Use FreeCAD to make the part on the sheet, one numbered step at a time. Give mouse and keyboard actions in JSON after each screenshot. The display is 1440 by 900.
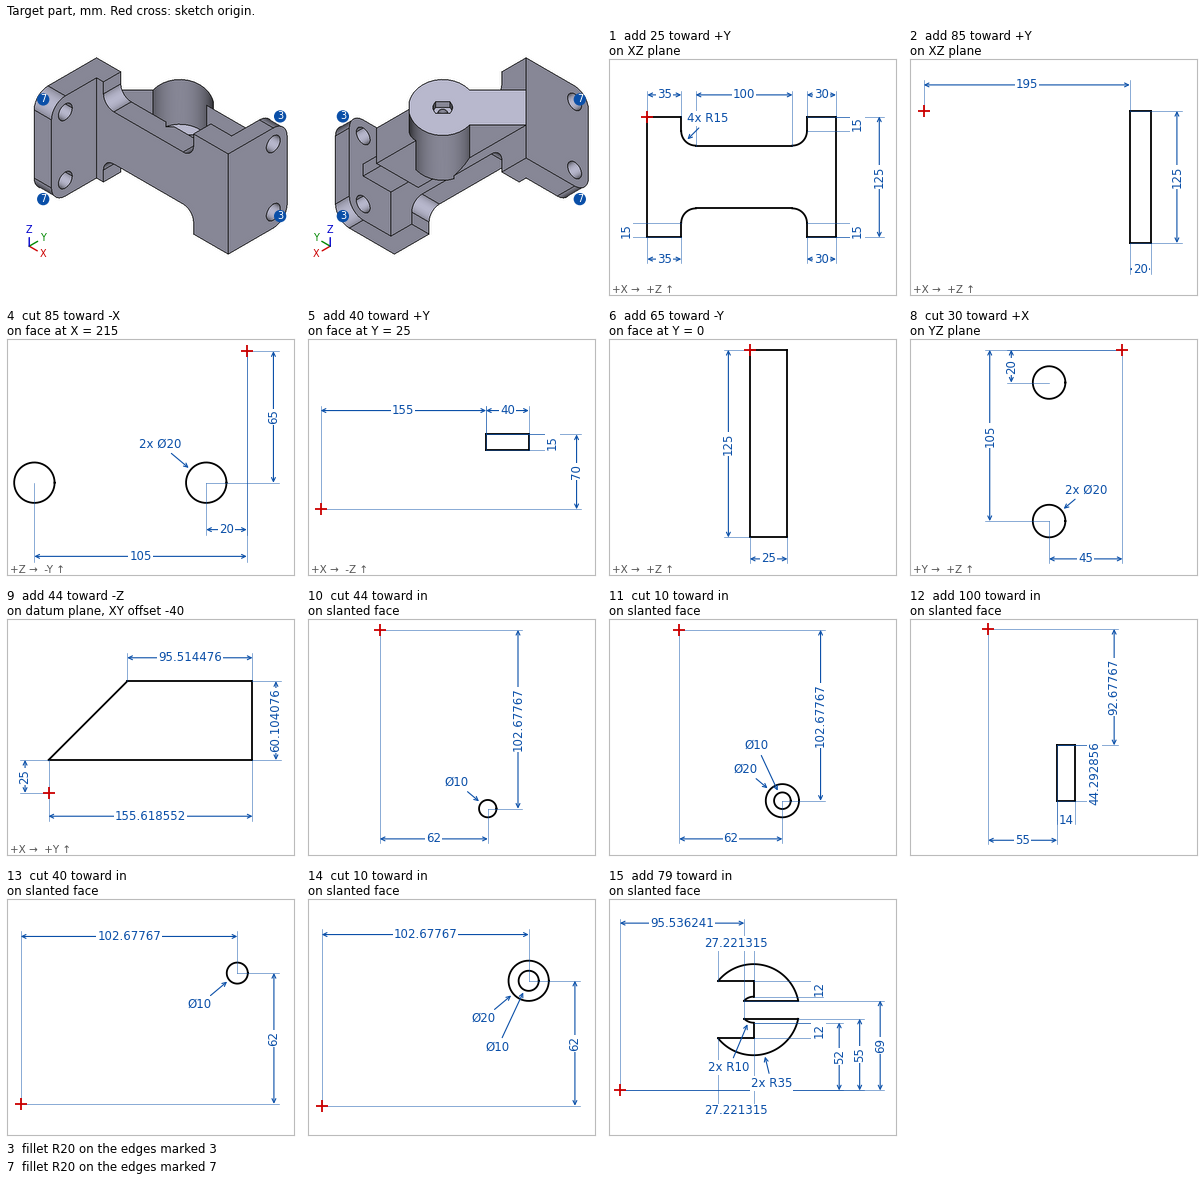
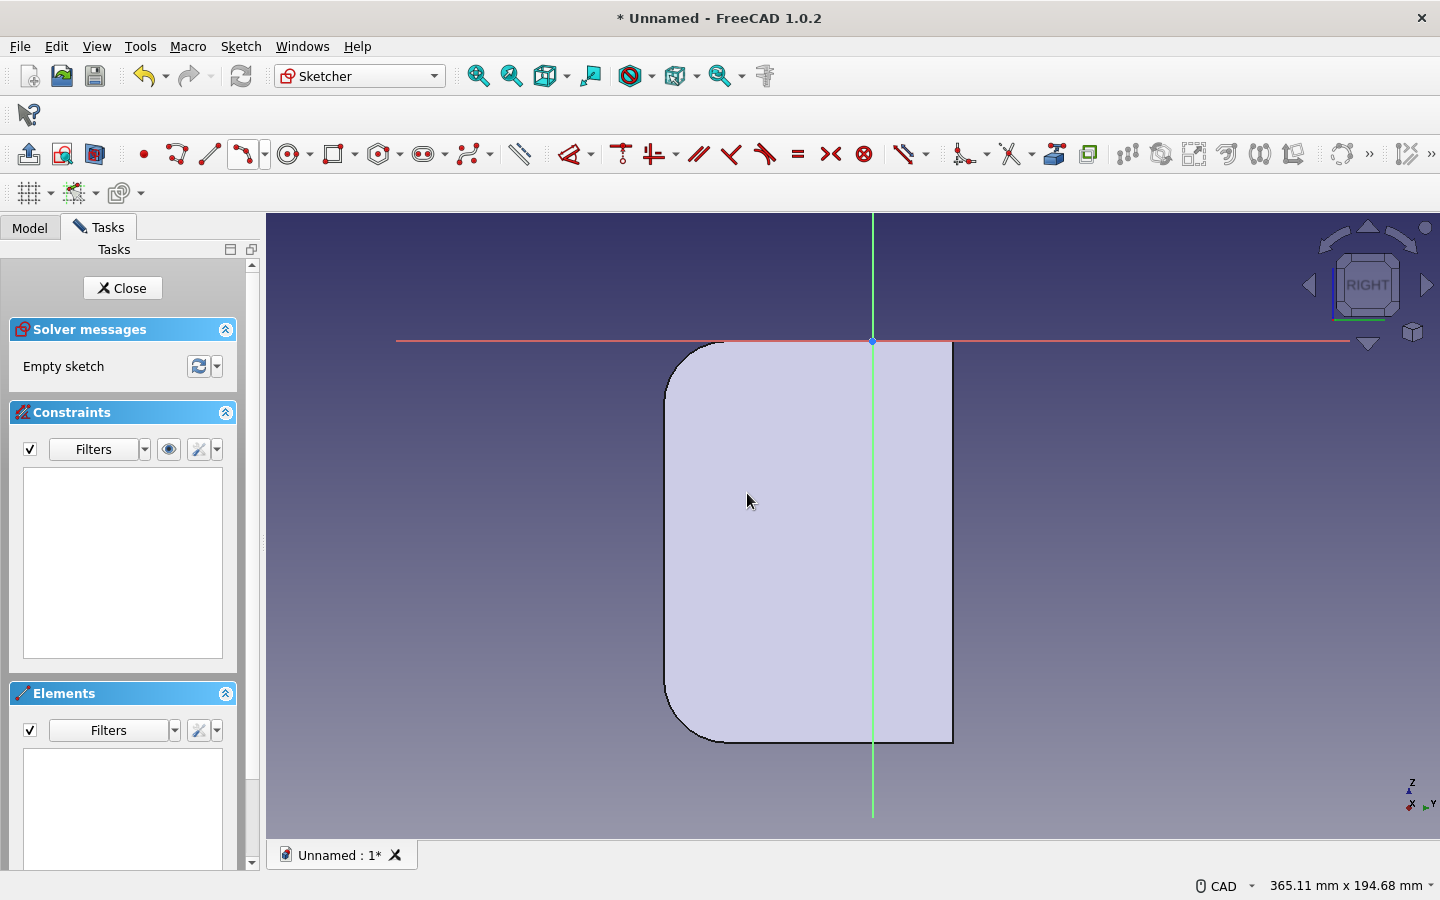
{"action": "key", "text": "g c"}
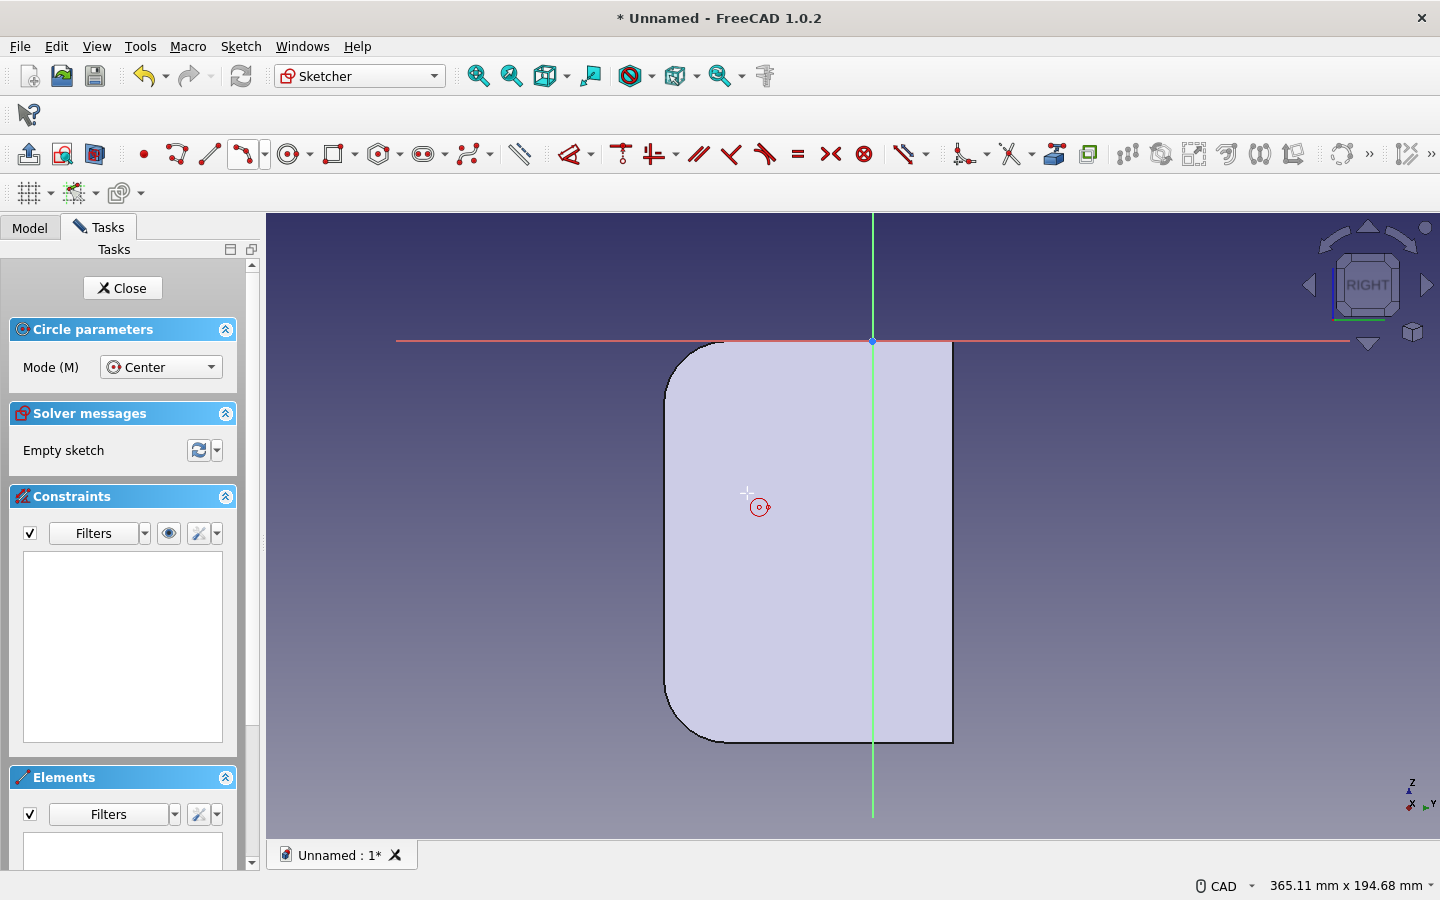
{"action": "left_click", "coordinate": [728, 679]}
{"action": "left_click", "coordinate": [751, 656]}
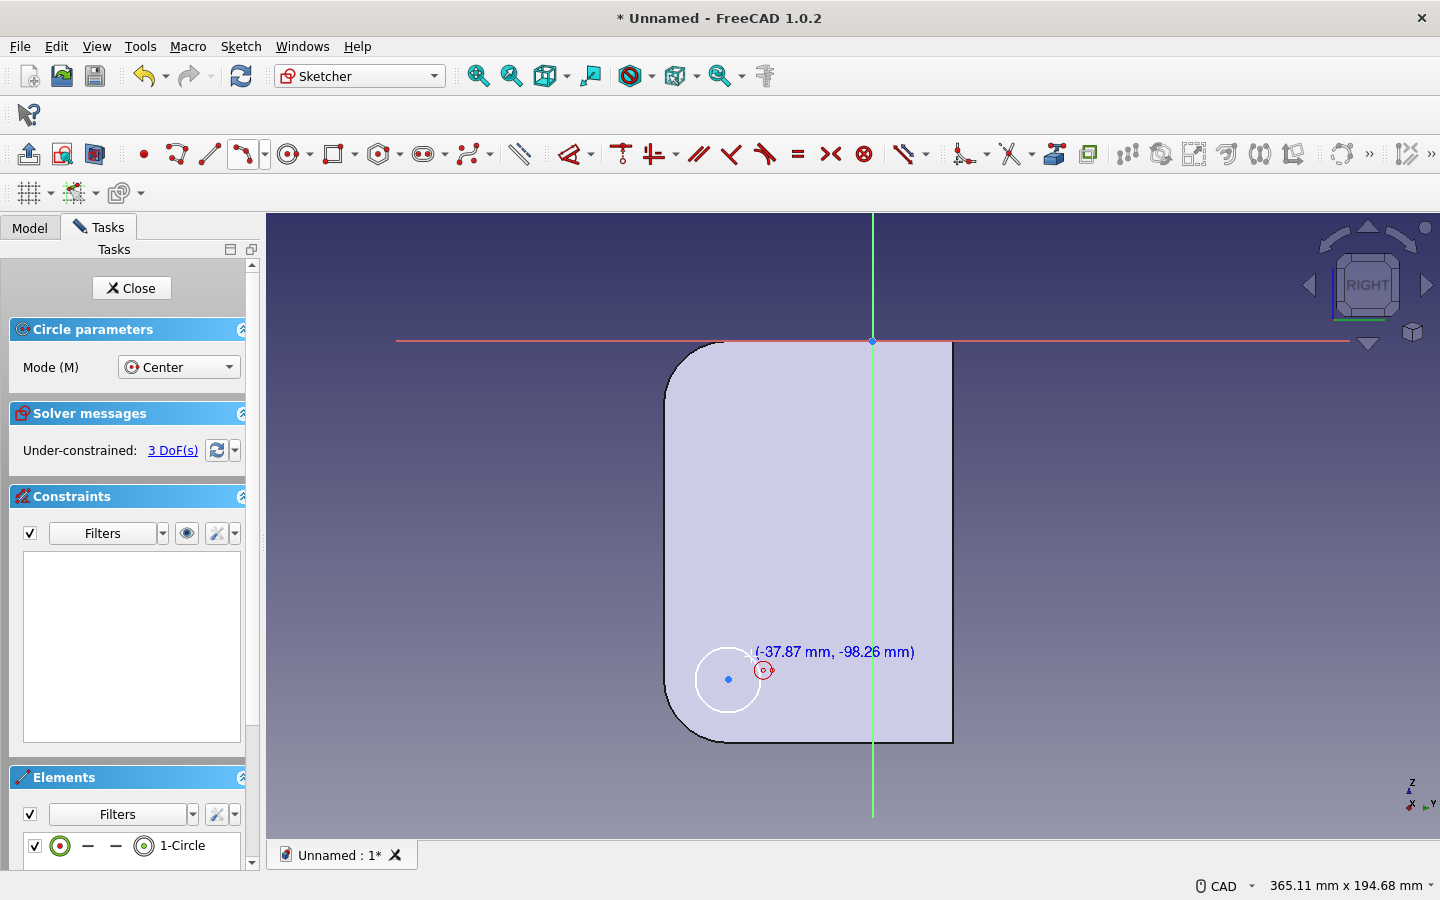
{"action": "left_click", "coordinate": [728, 405]}
{"action": "left_click", "coordinate": [751, 383]}
{"action": "key", "text": "Escape"}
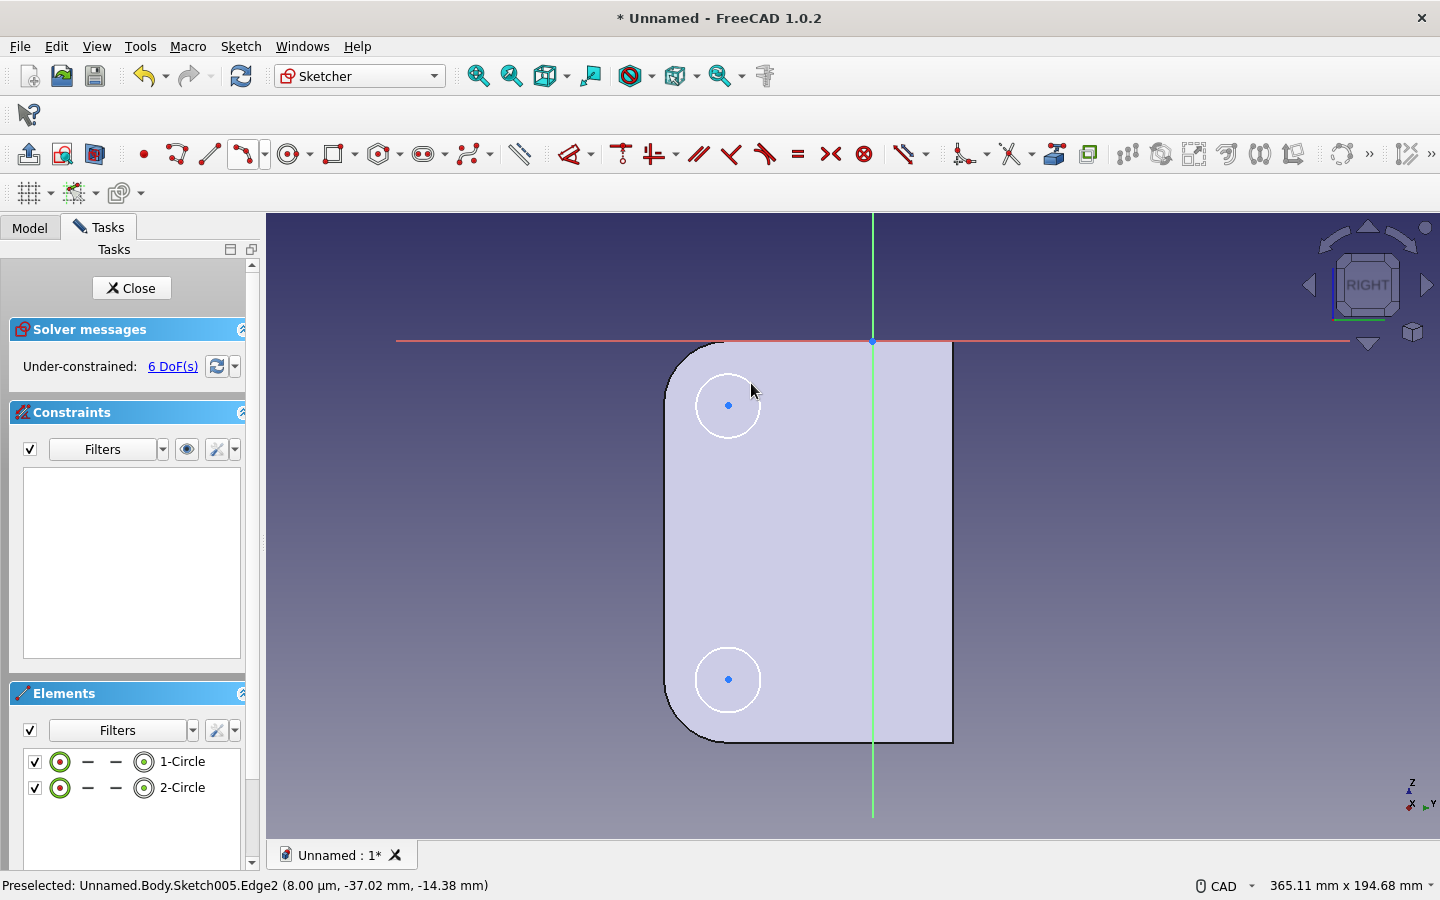
{"action": "left_click", "coordinate": [751, 657]}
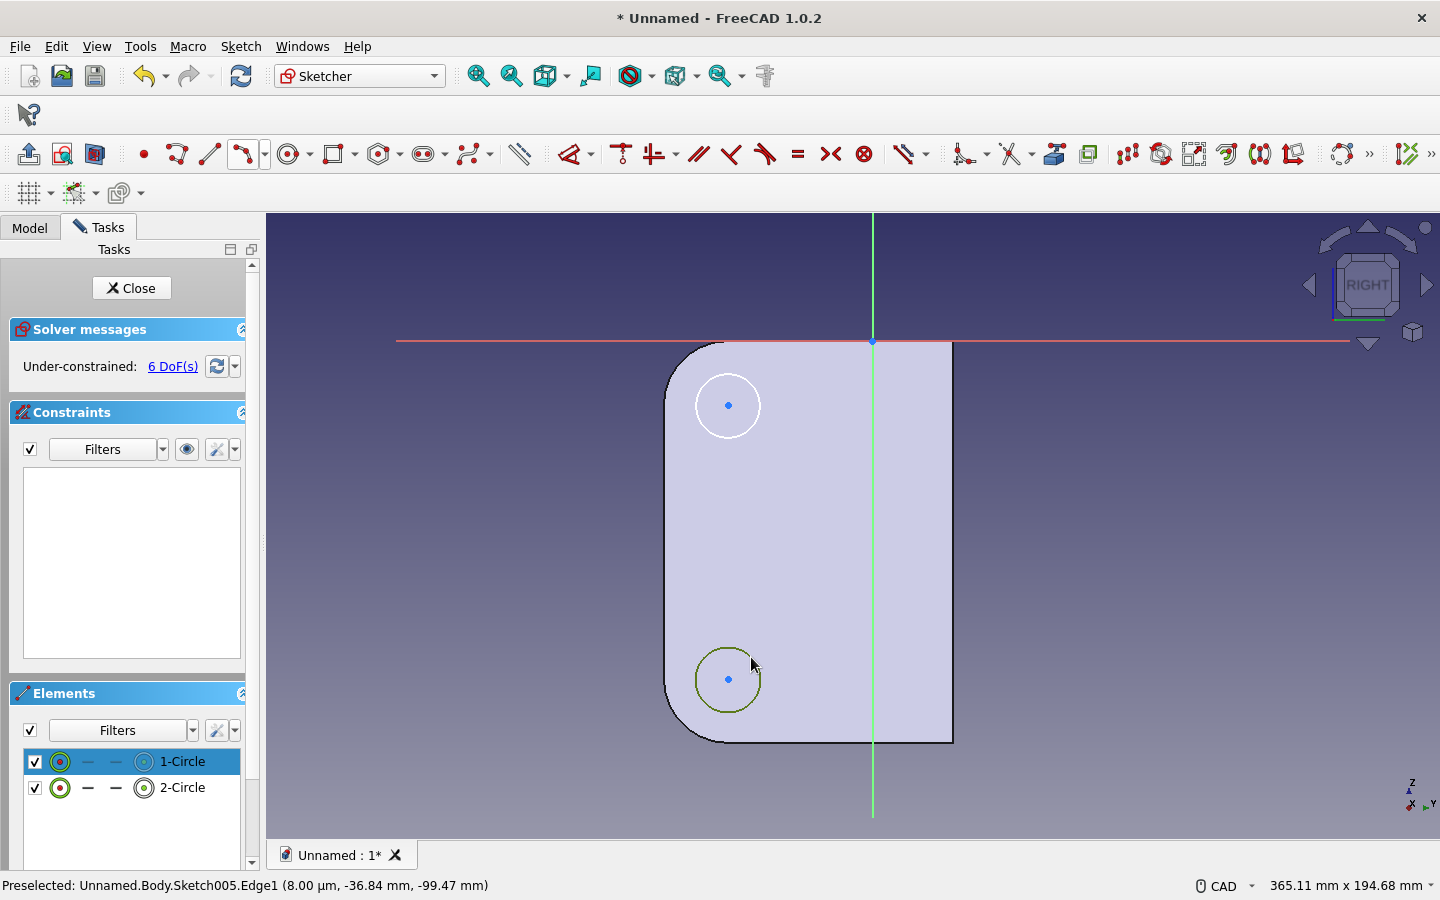
{"action": "left_click", "coordinate": [750, 383]}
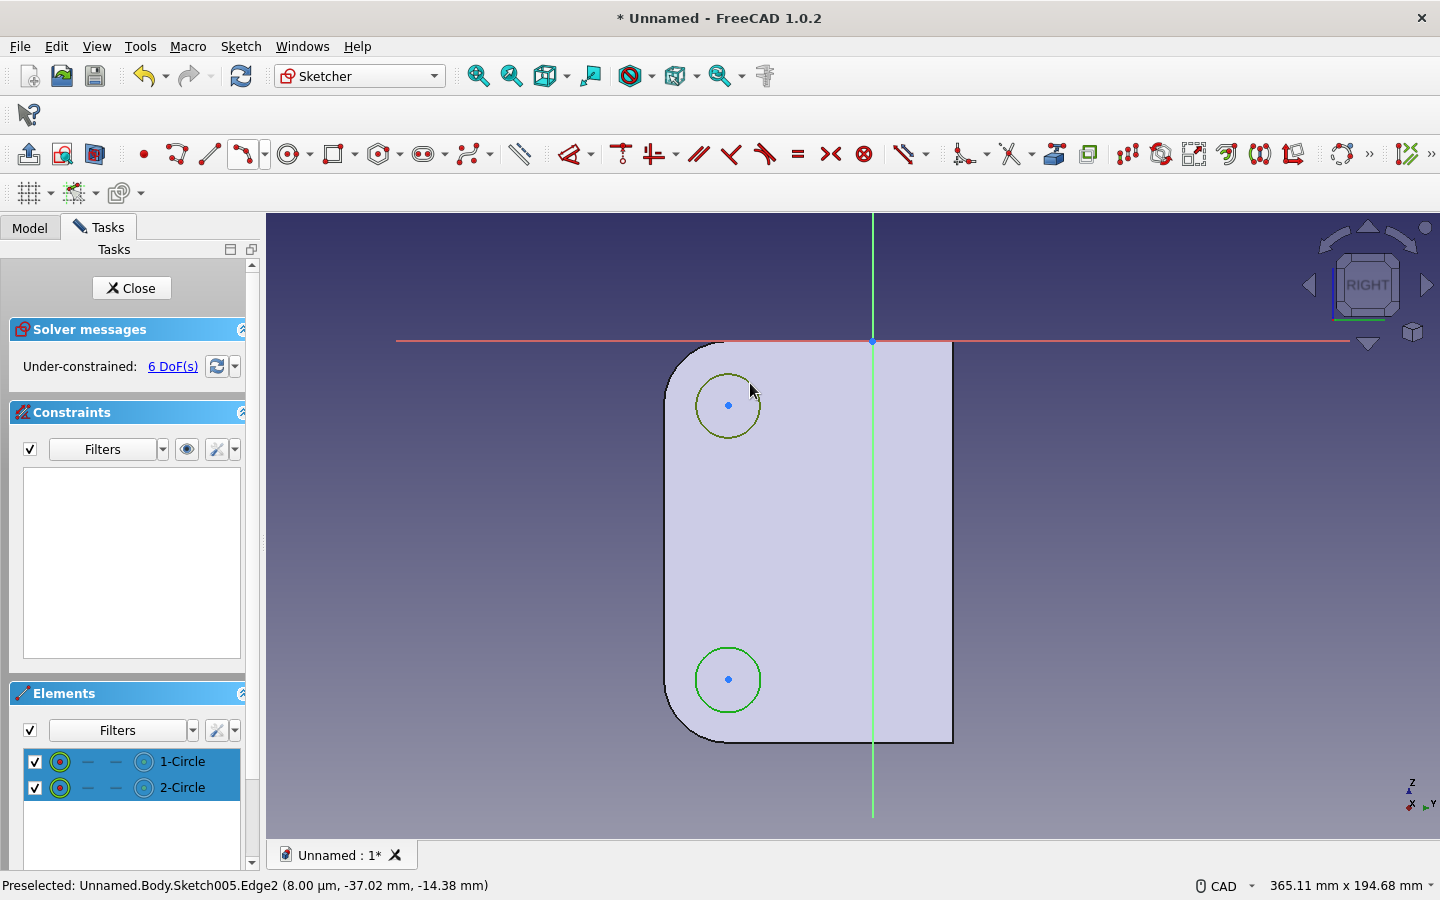
{"action": "left_click", "coordinate": [798, 154]}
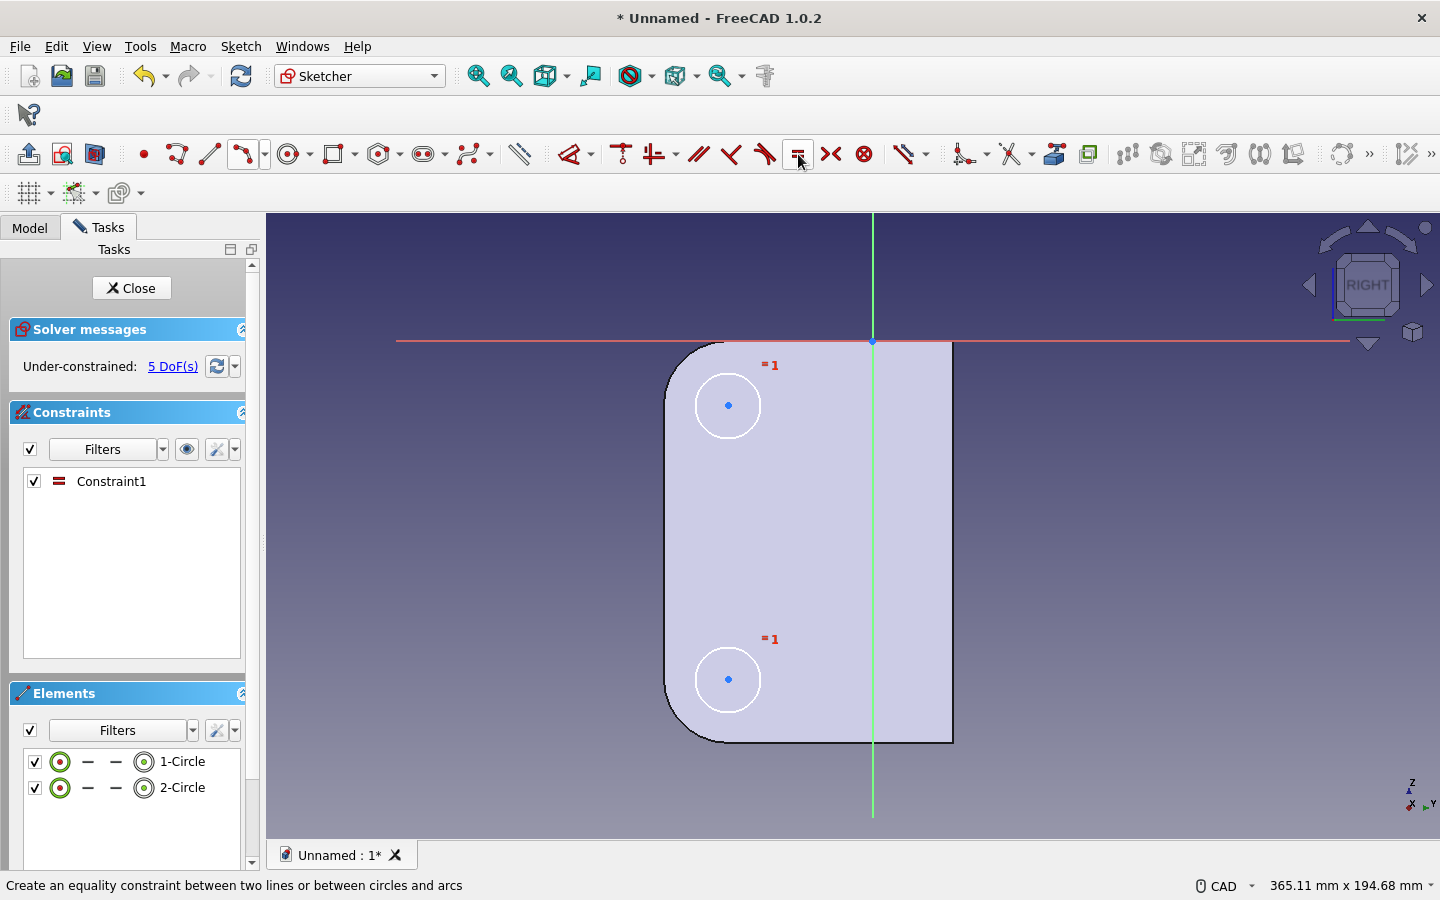
{"action": "left_click", "coordinate": [728, 680]}